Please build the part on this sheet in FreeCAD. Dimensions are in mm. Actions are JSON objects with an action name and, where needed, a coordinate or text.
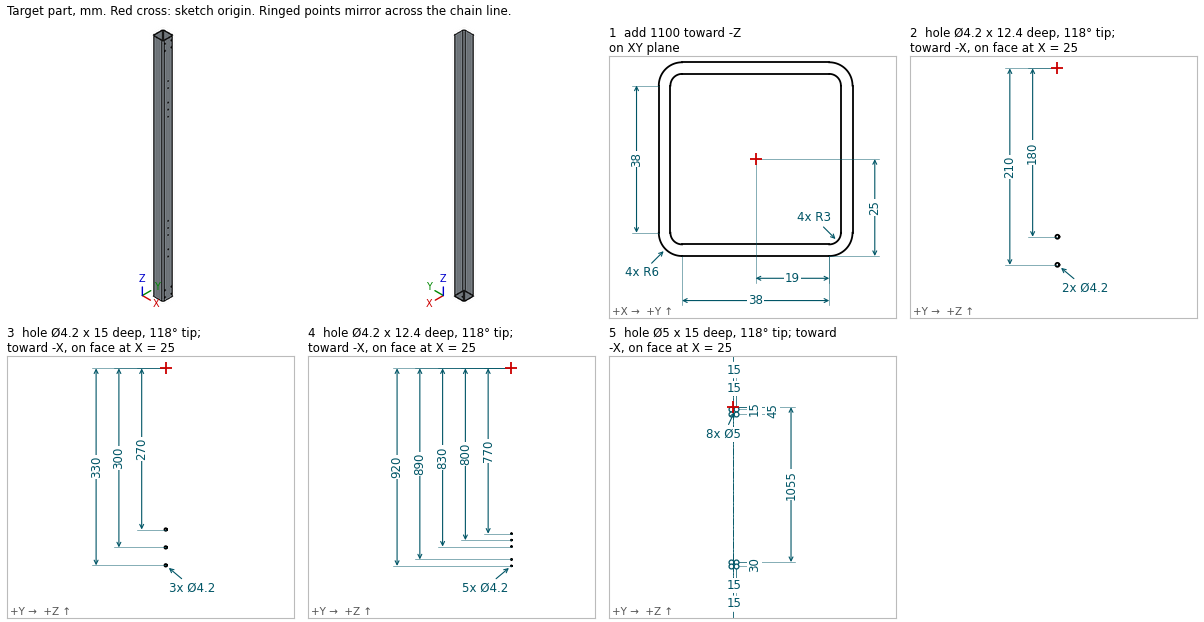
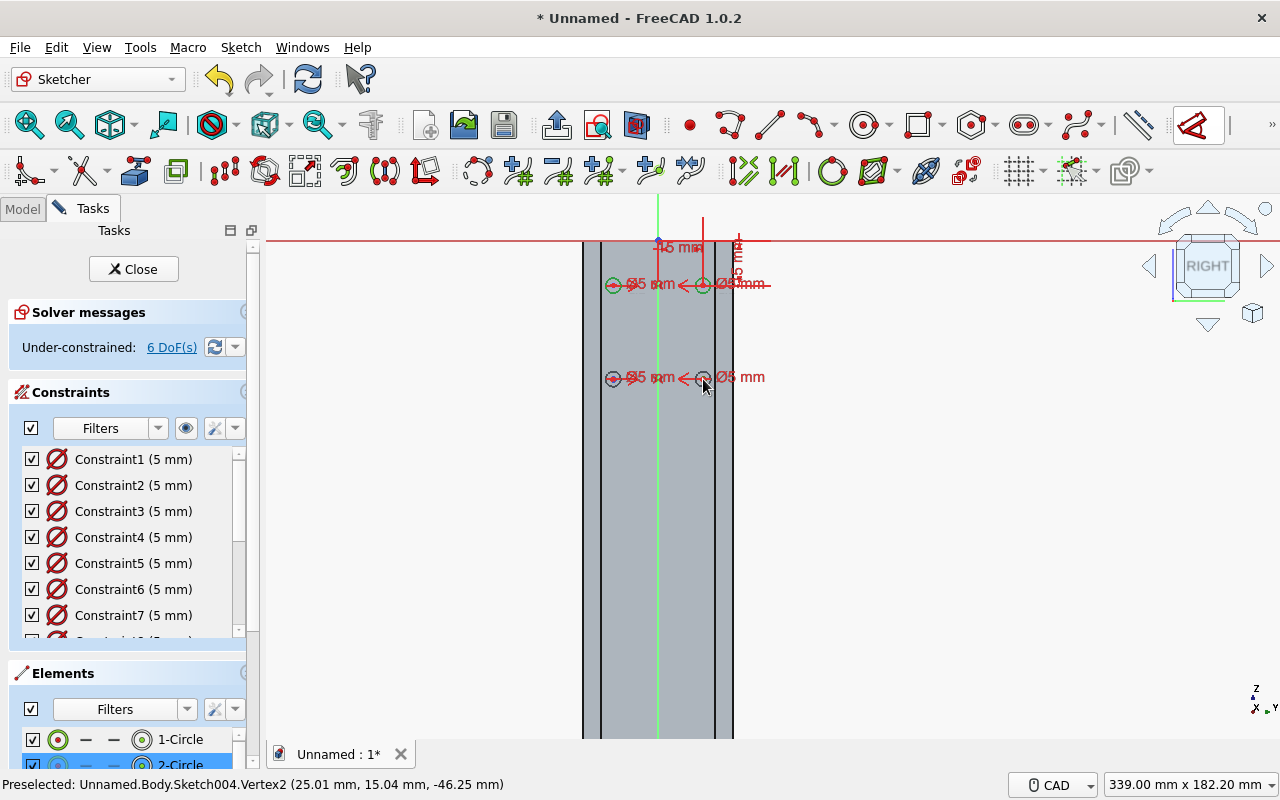
{"action": "left_click", "coordinate": [1218, 126]}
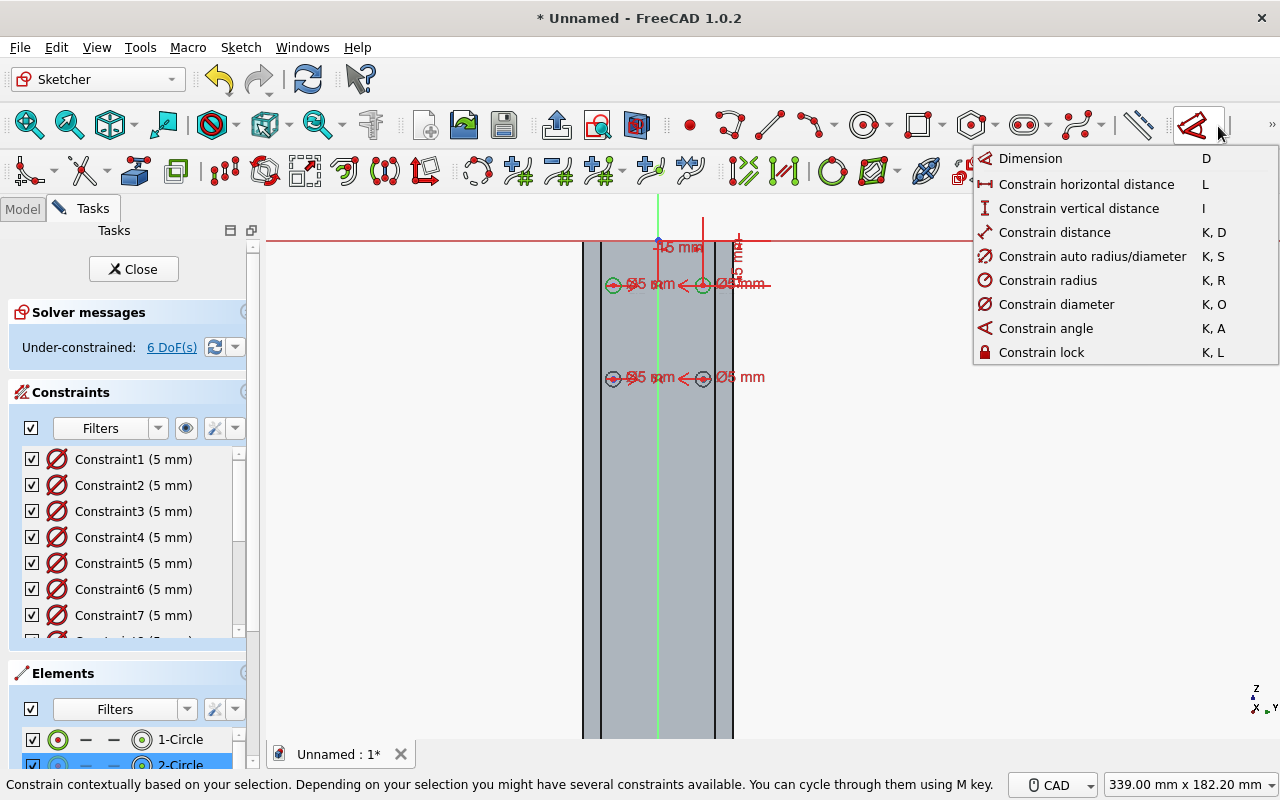
{"action": "left_click", "coordinate": [1126, 184]}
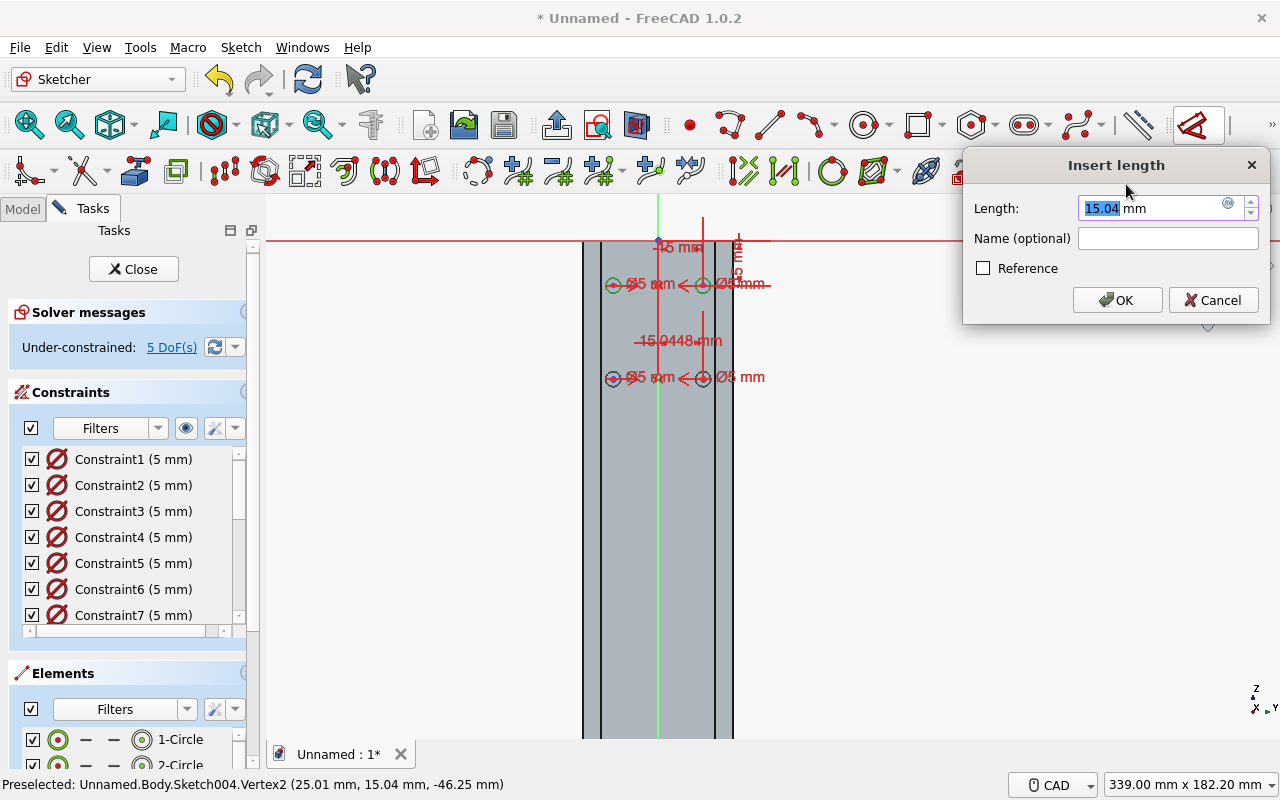
{"action": "type", "text": "15"}
{"action": "key", "text": "Return"}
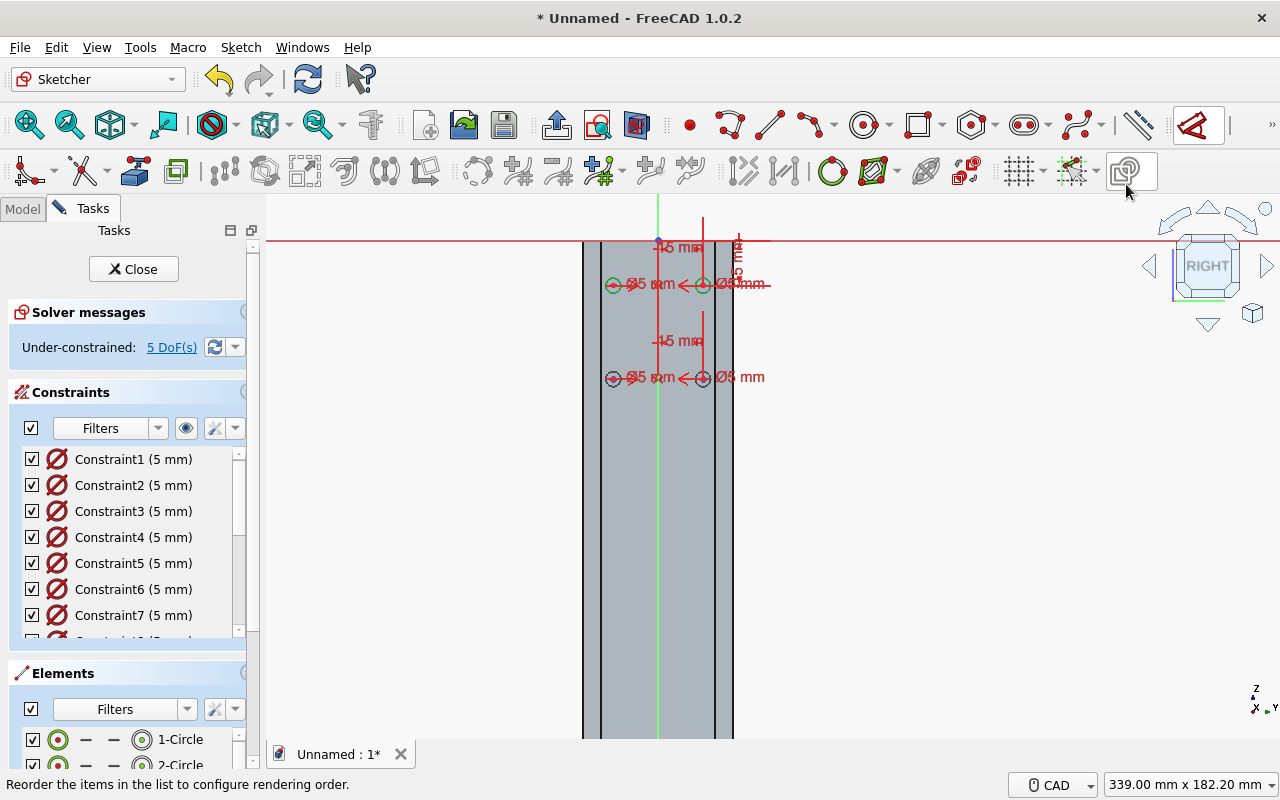
{"action": "scroll", "coordinate": [710, 292], "scroll_direction": "down", "scroll_amount": 11}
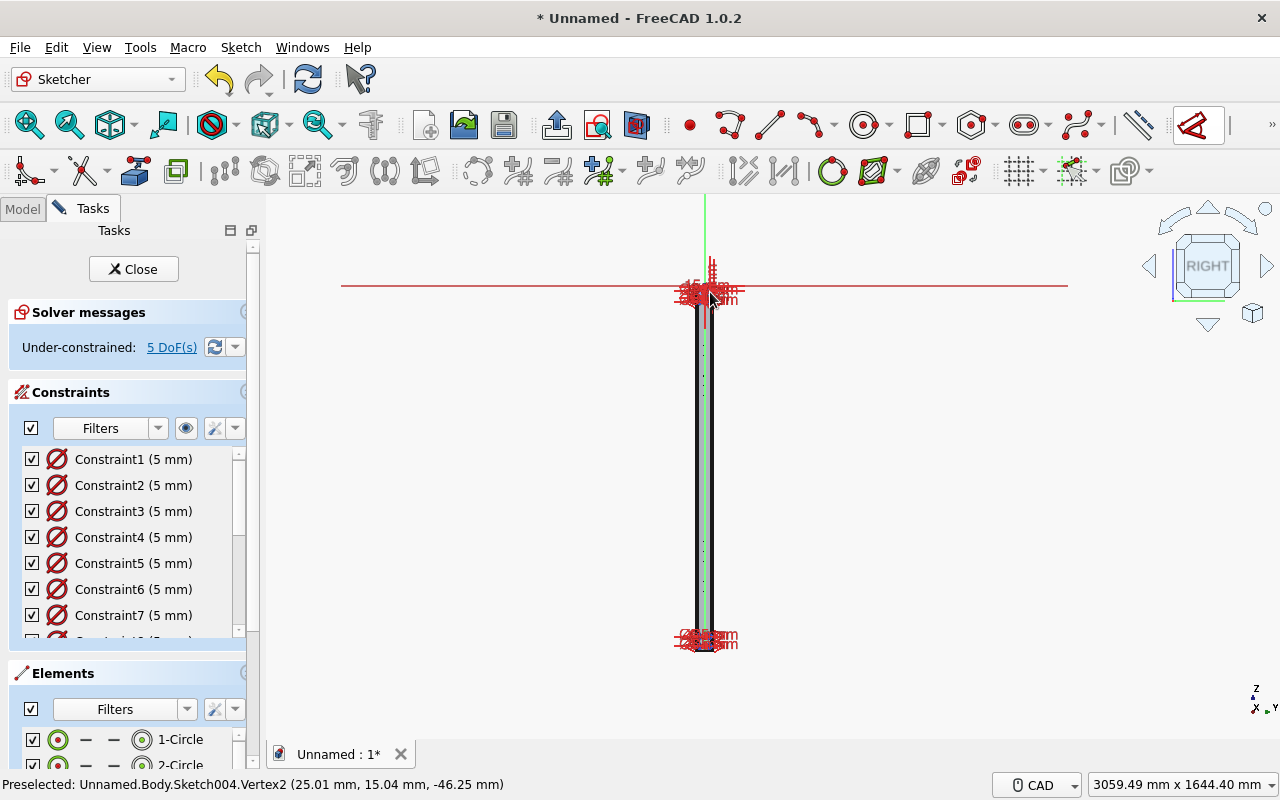
{"action": "scroll", "coordinate": [710, 302], "scroll_direction": "up", "scroll_amount": 5}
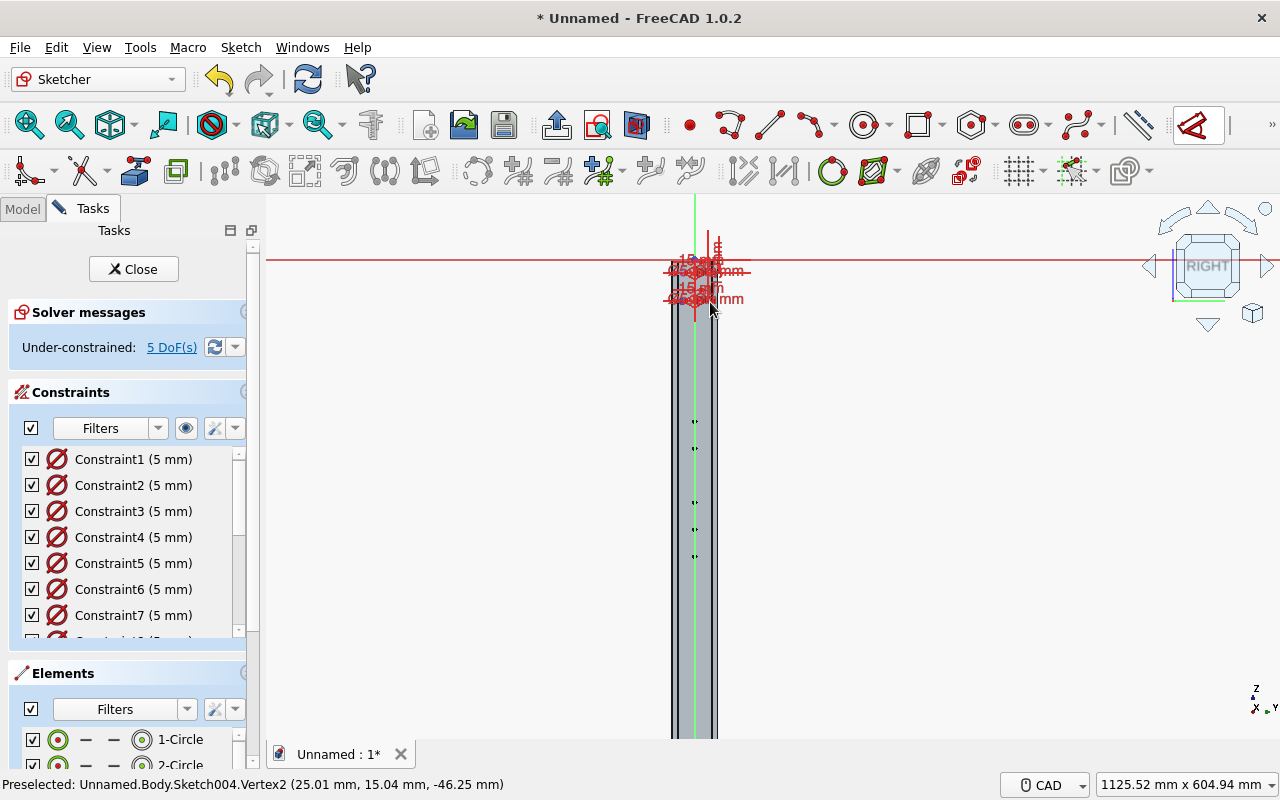
{"action": "left_click", "coordinate": [708, 301]}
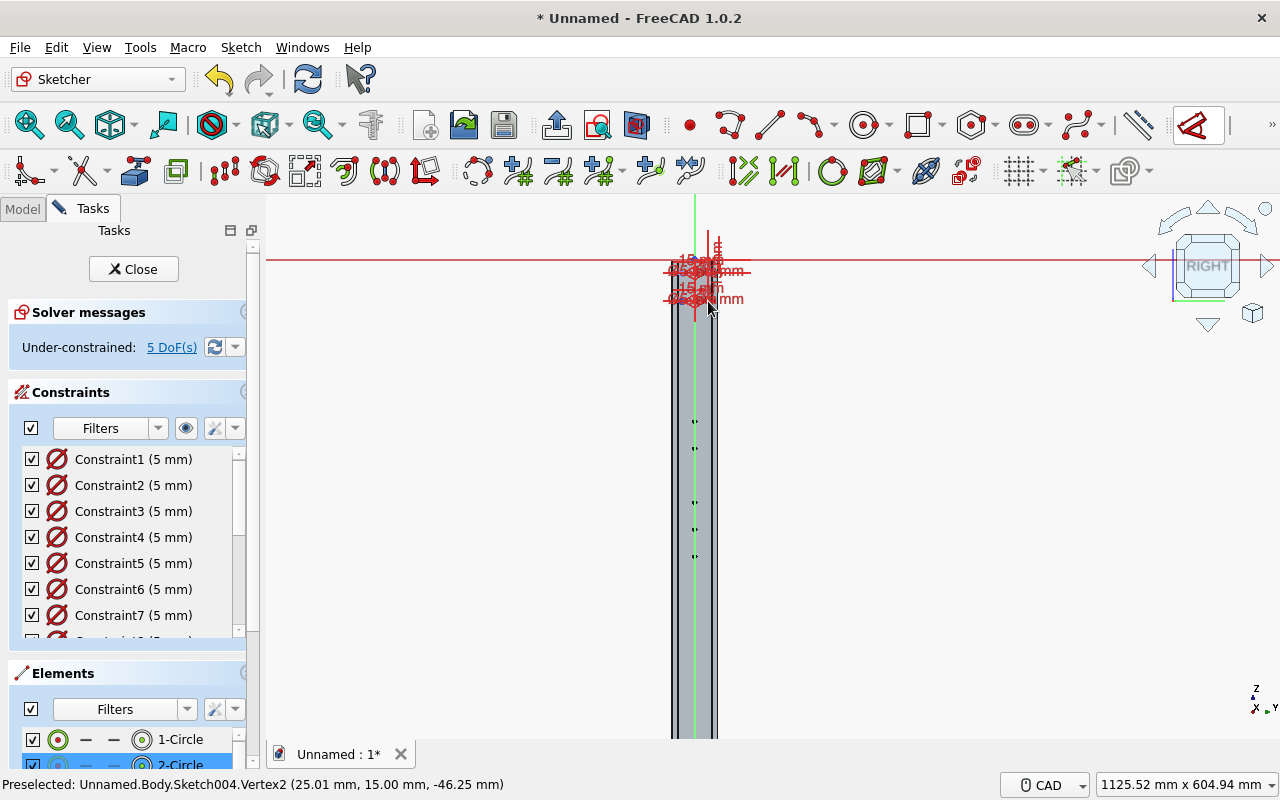
{"action": "key", "text": "i"}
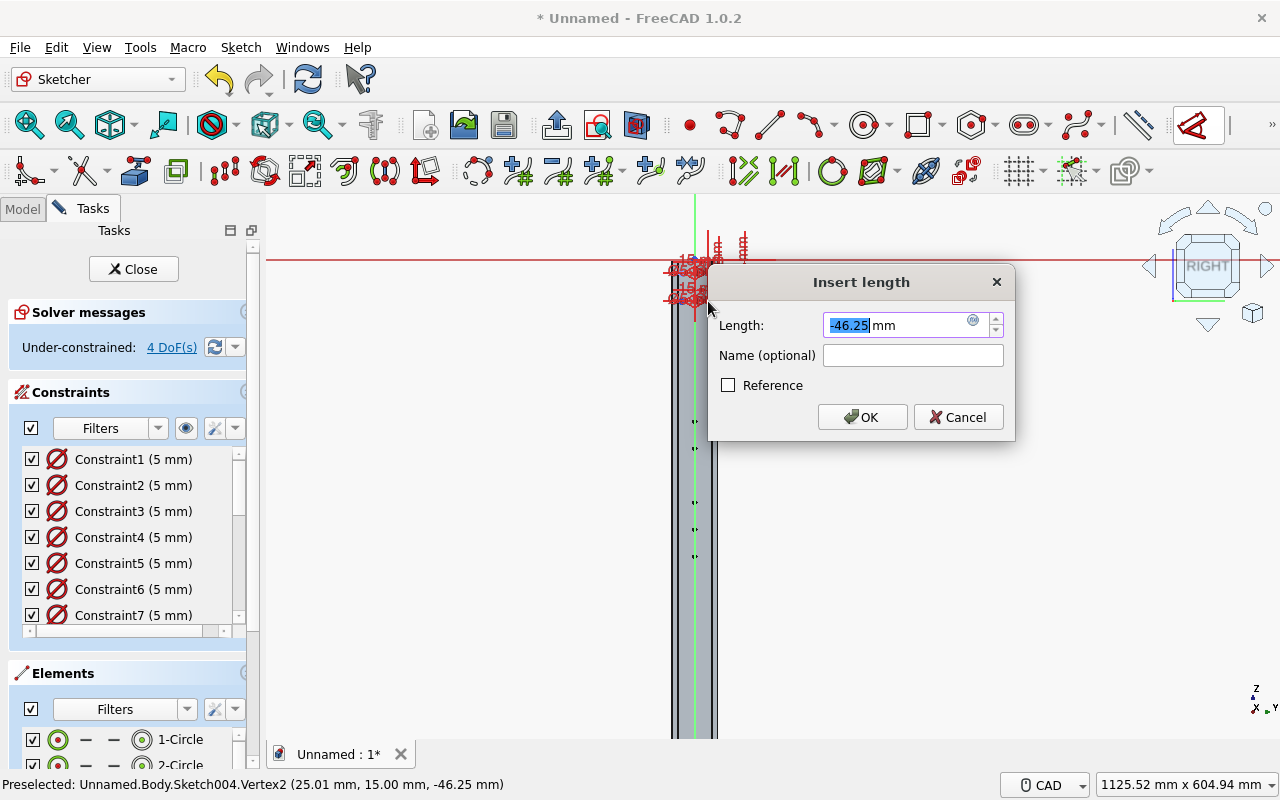
{"action": "type", "text": "-45"}
{"action": "key", "text": "Return"}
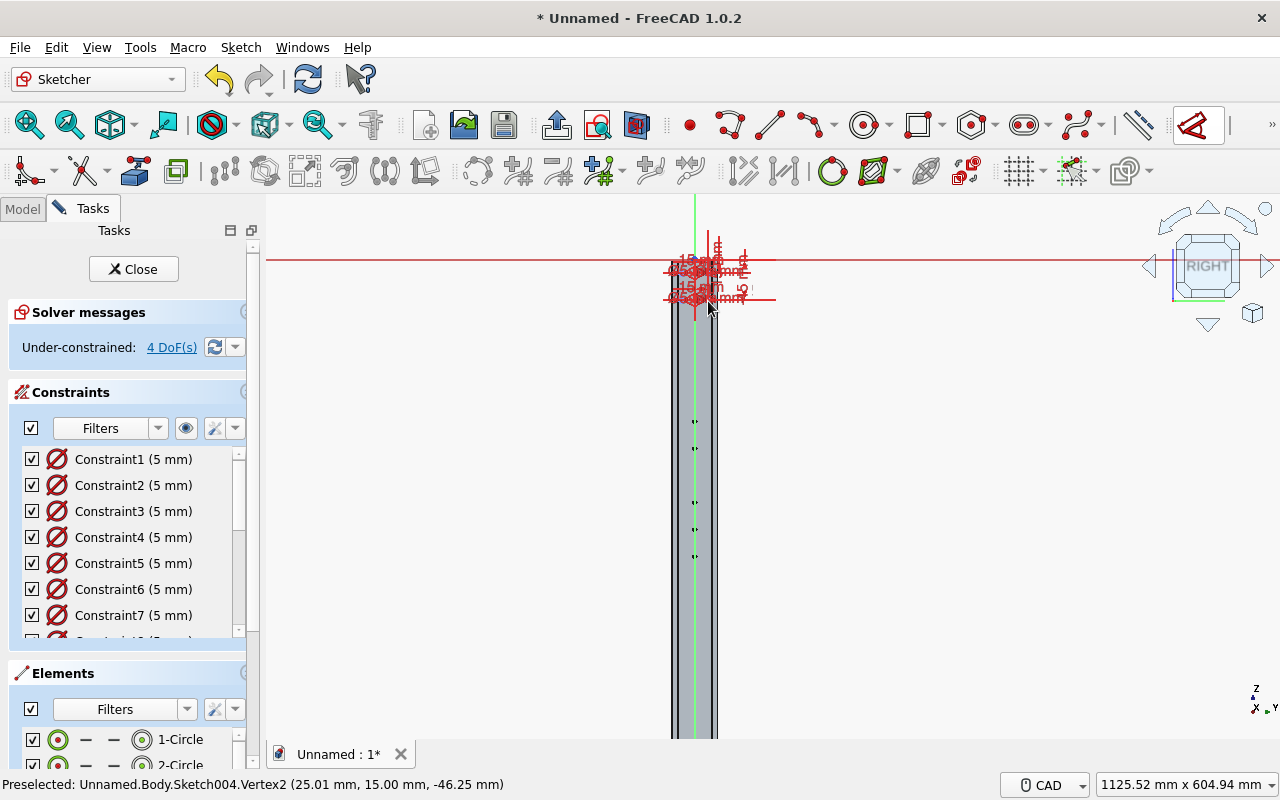
{"action": "scroll", "coordinate": [710, 302], "scroll_direction": "down", "scroll_amount": 5}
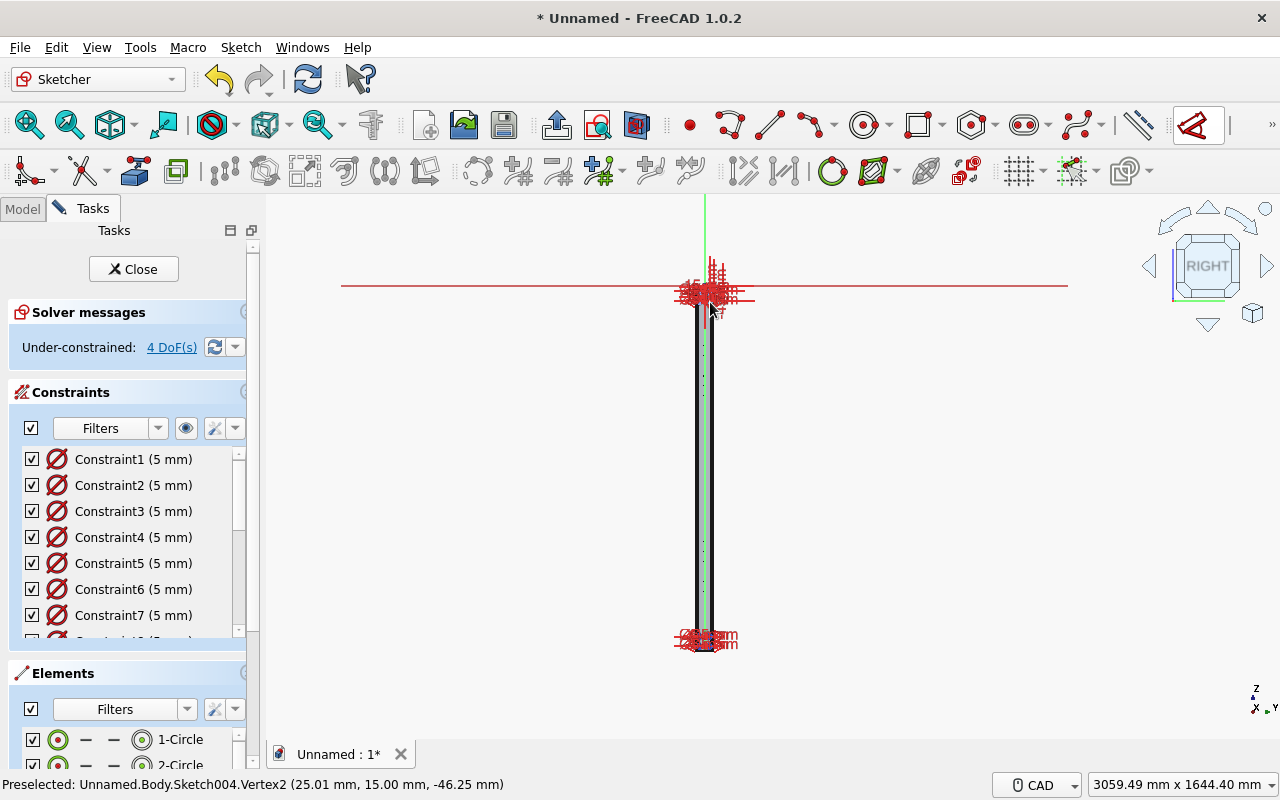
{"action": "scroll", "coordinate": [710, 637], "scroll_direction": "up", "scroll_amount": 11}